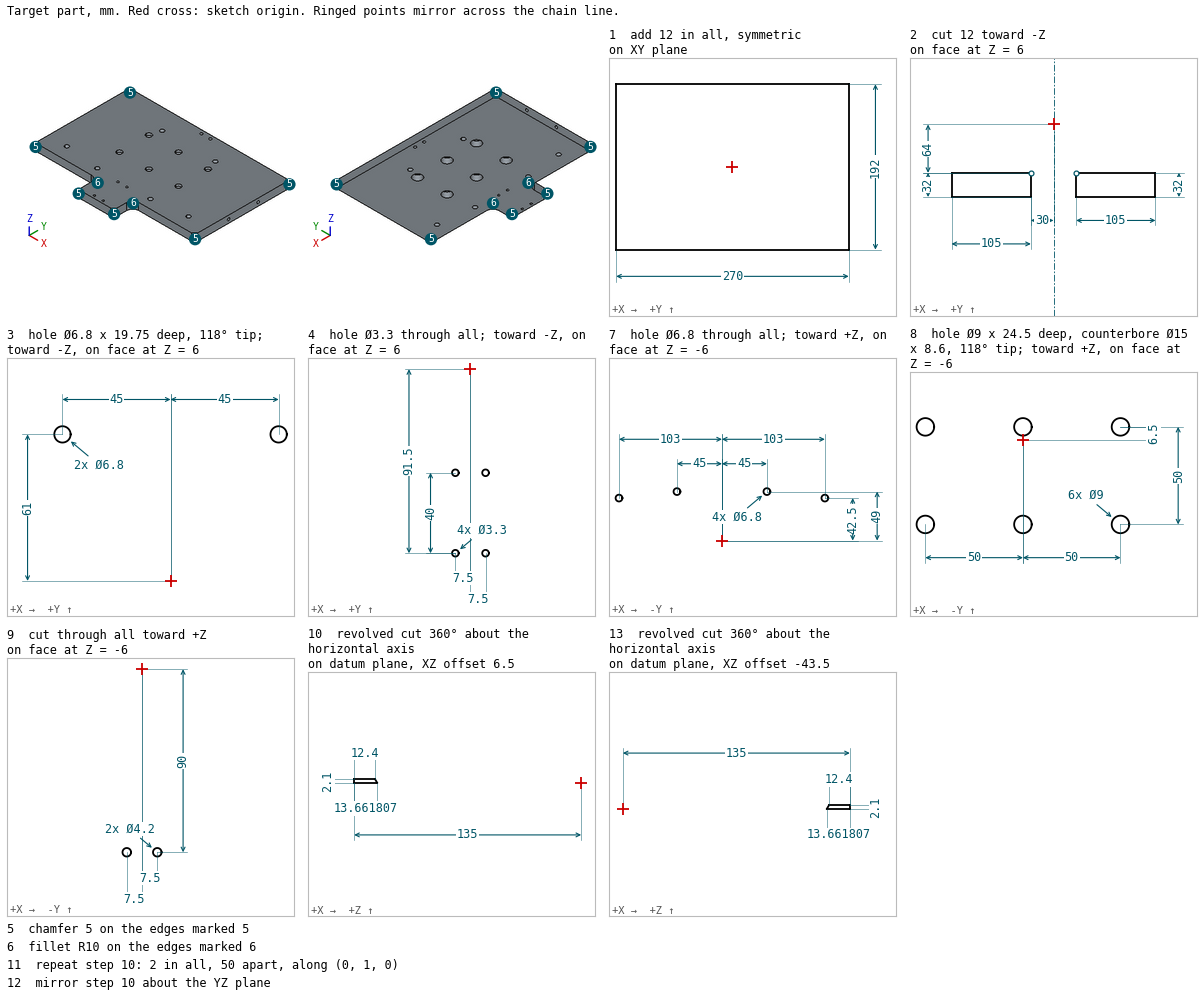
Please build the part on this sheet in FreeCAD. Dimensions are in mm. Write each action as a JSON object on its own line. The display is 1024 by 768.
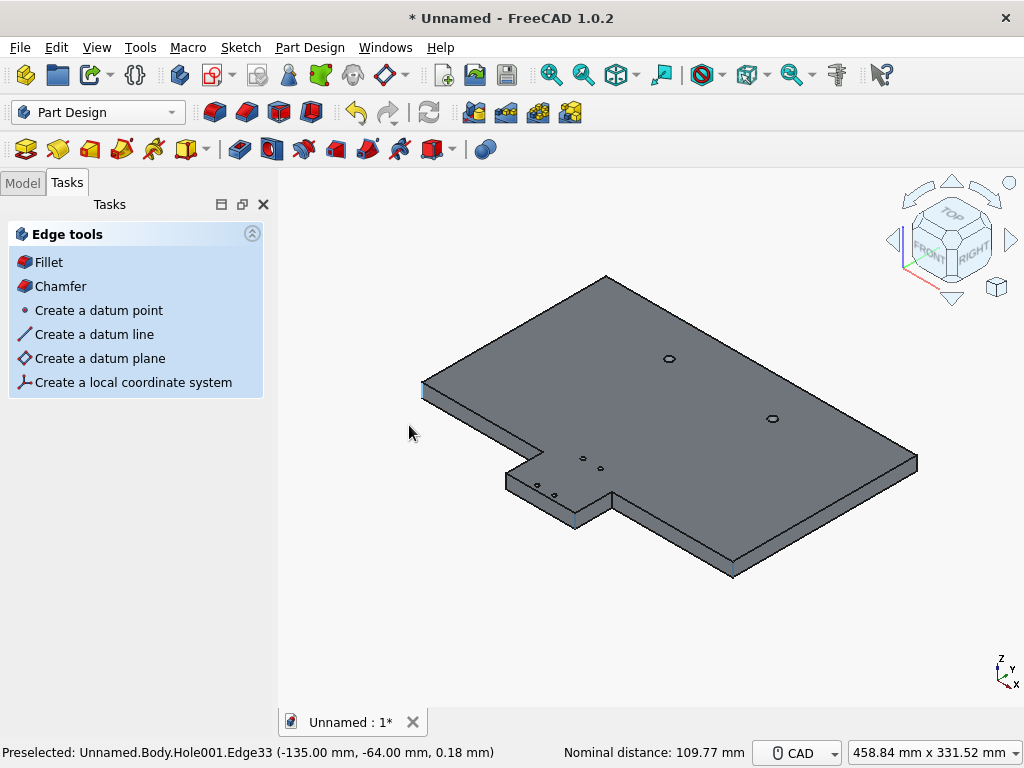
{"action": "scroll", "coordinate": [422, 389], "scroll_direction": "up", "scroll_amount": 4}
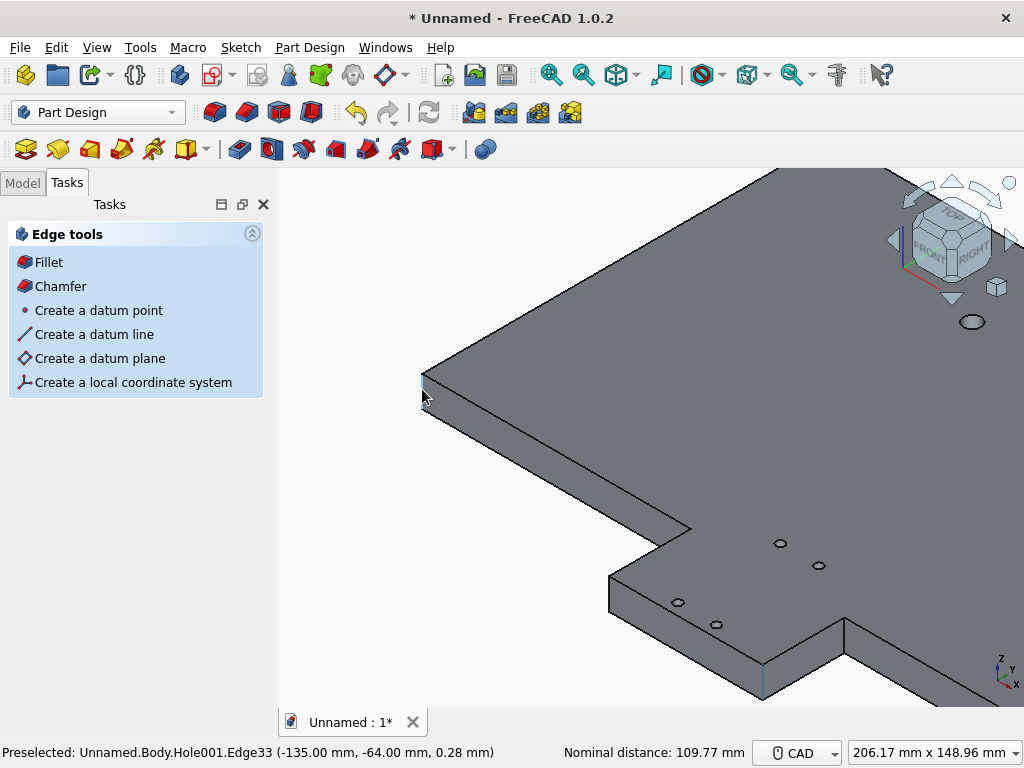
{"action": "key", "text": "v f"}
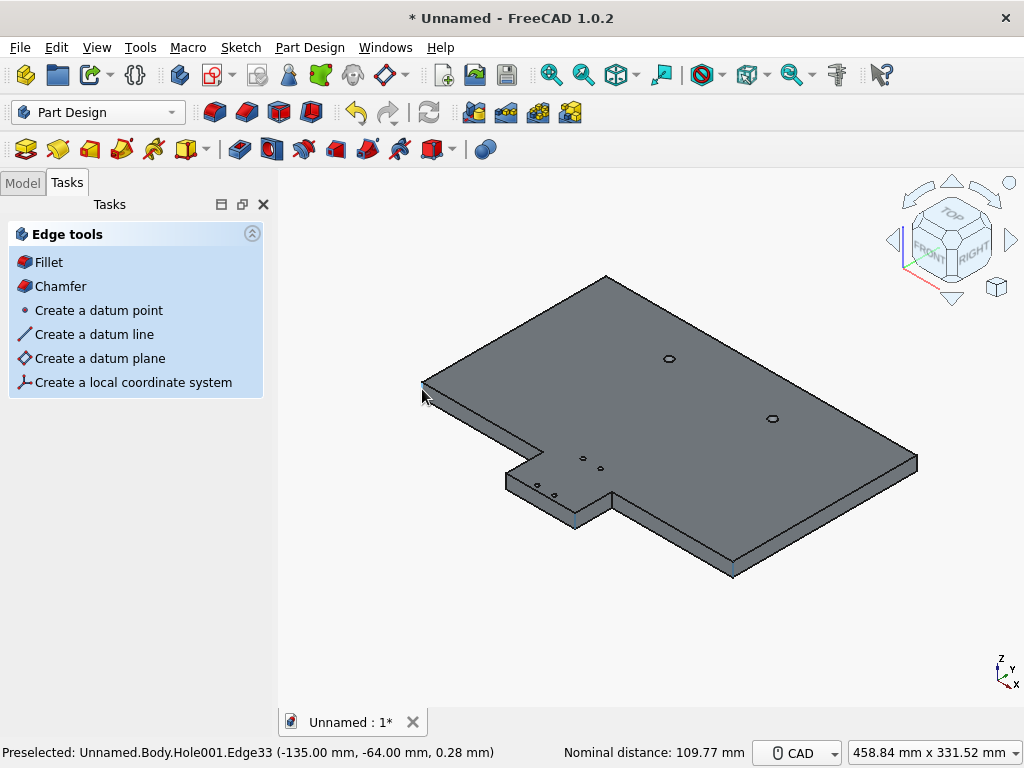
{"action": "key", "text": "2"}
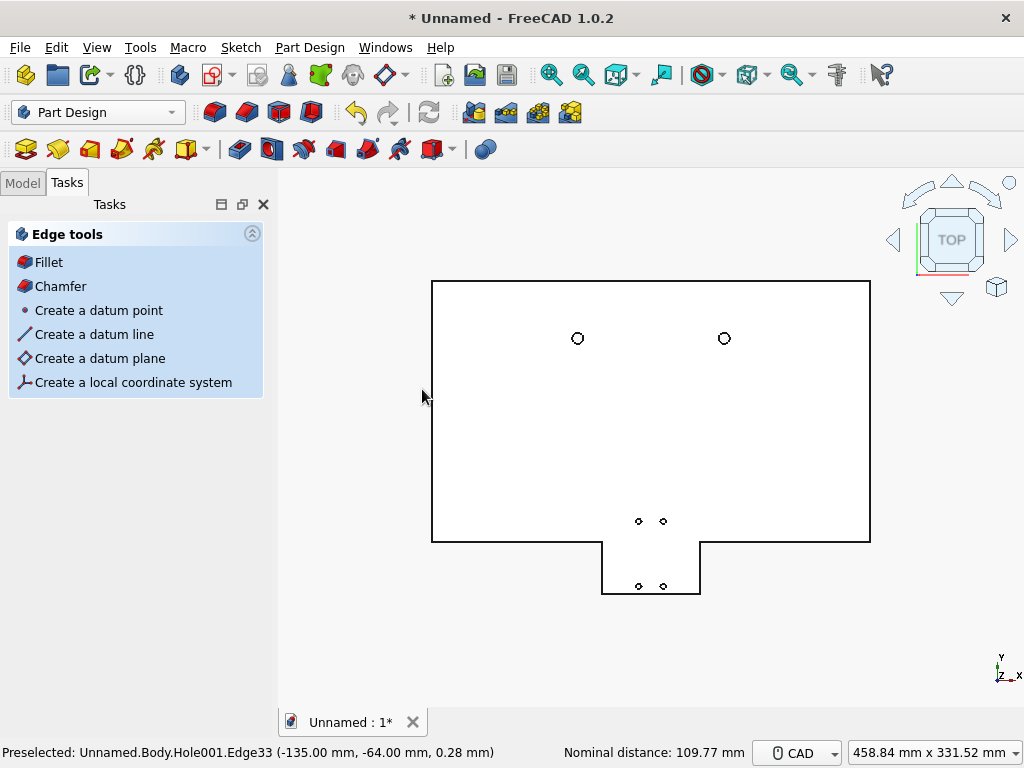
{"action": "scroll", "coordinate": [432, 541], "scroll_direction": "up", "scroll_amount": 4}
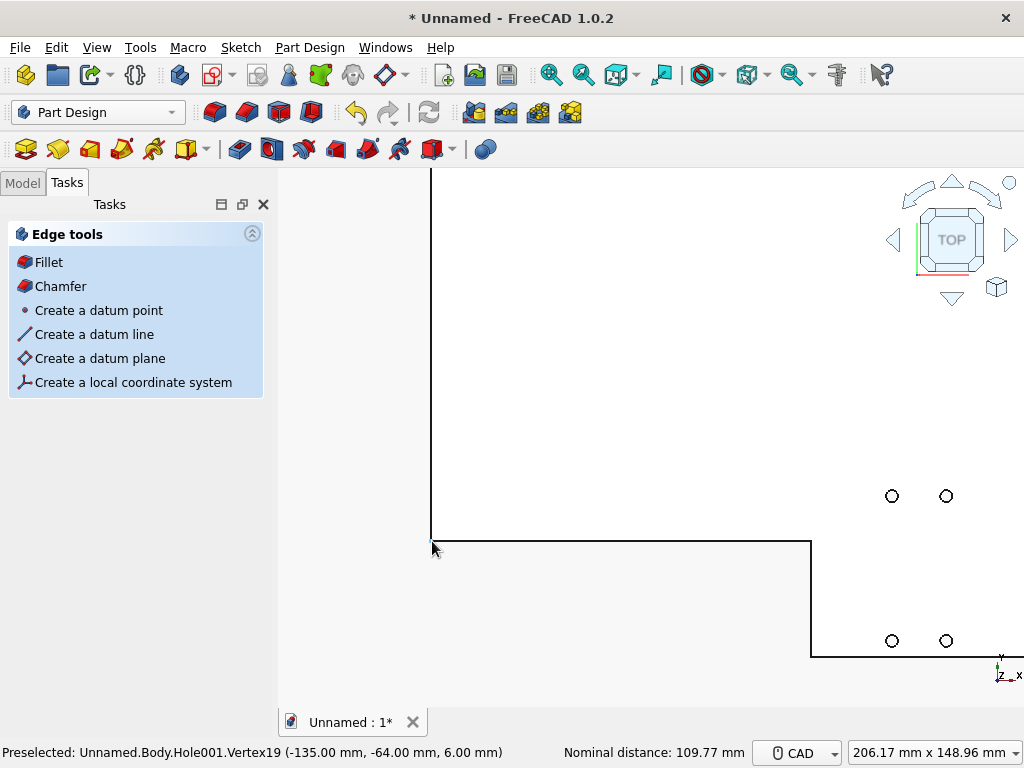
{"action": "key", "text": "v f"}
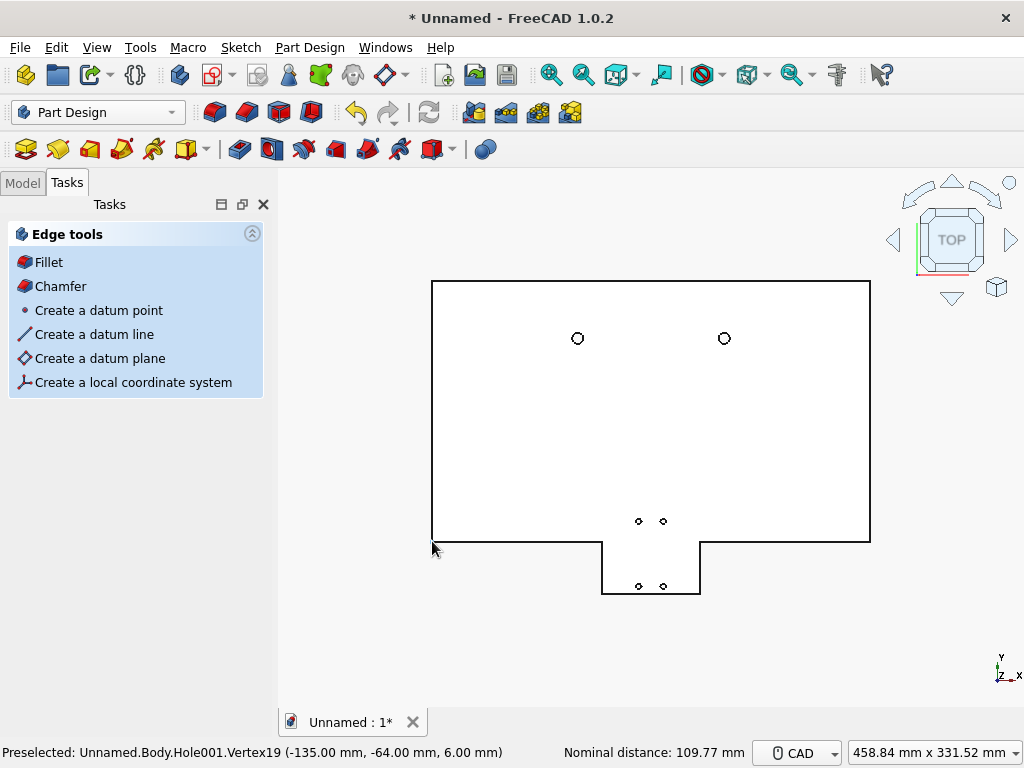
{"action": "key", "text": "1"}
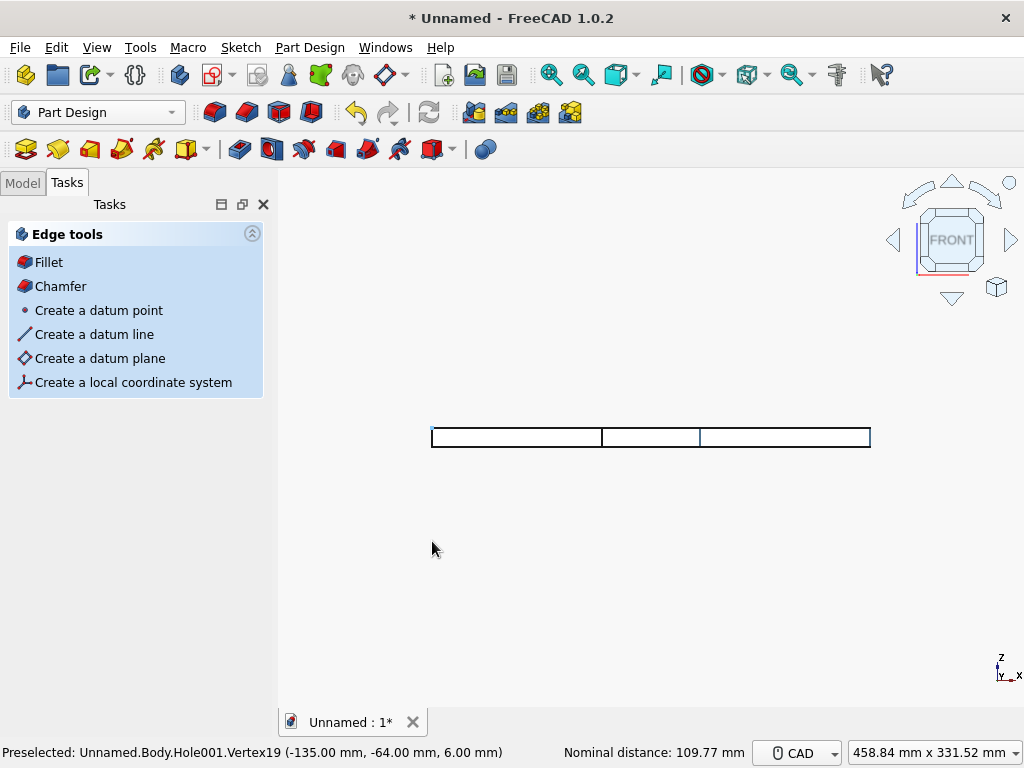
{"action": "left_click", "coordinate": [432, 436], "text": "ctrl"}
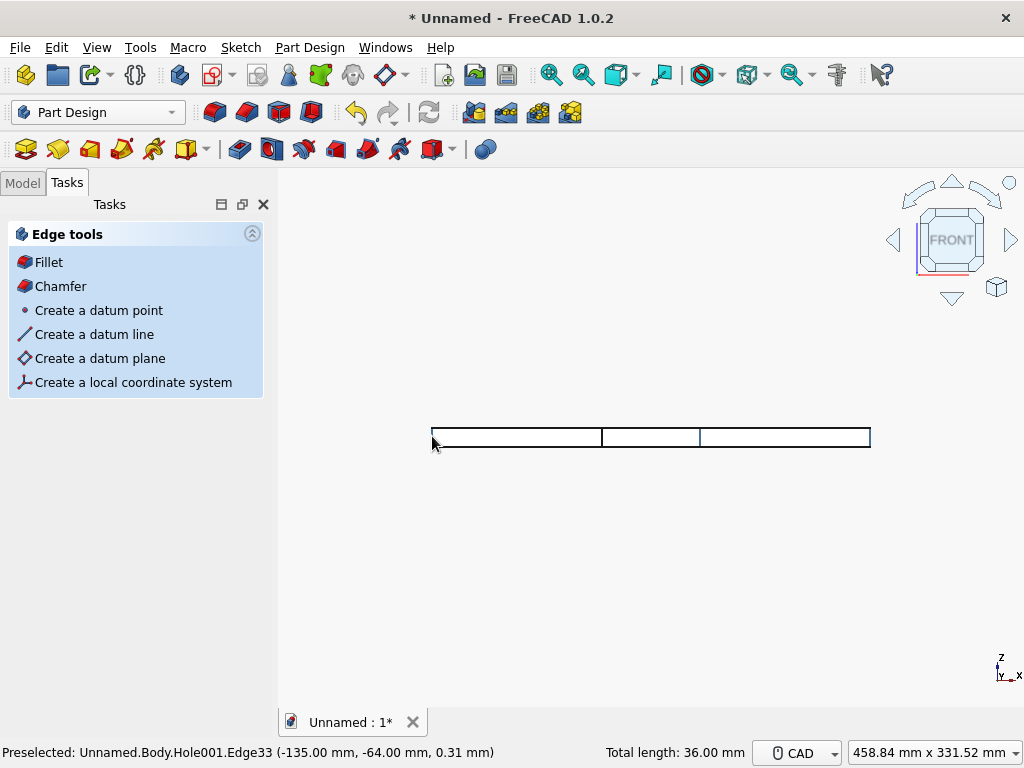
{"action": "left_click", "coordinate": [602, 436], "text": "ctrl"}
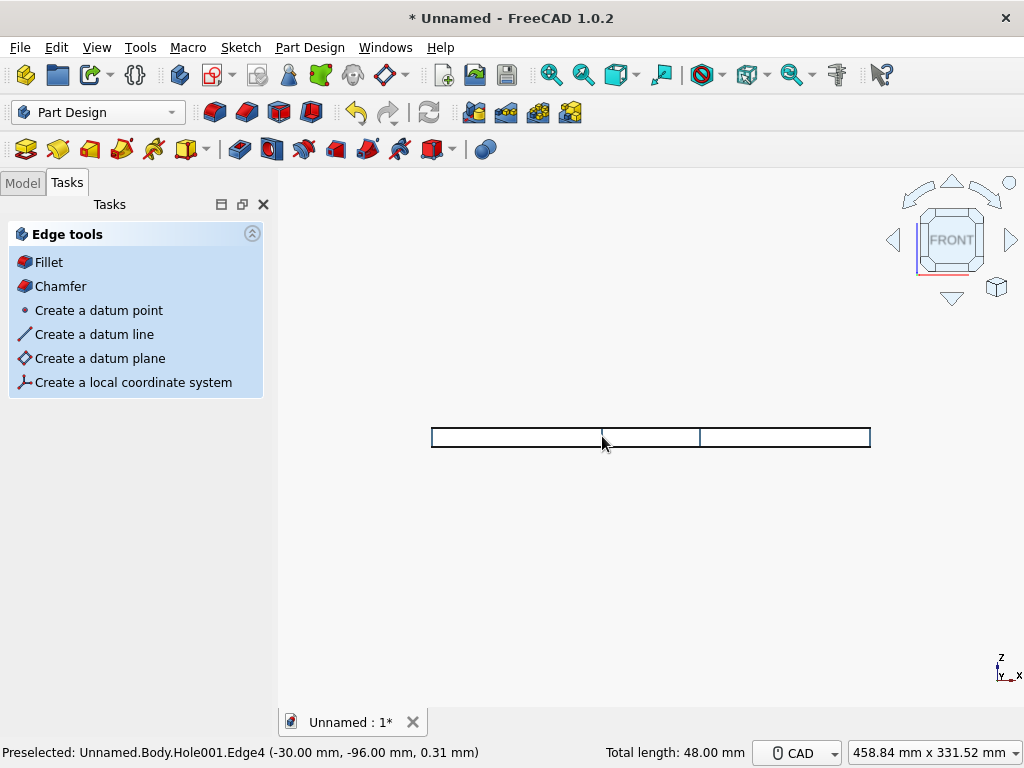
{"action": "scroll", "coordinate": [432, 436], "scroll_direction": "up", "scroll_amount": 4}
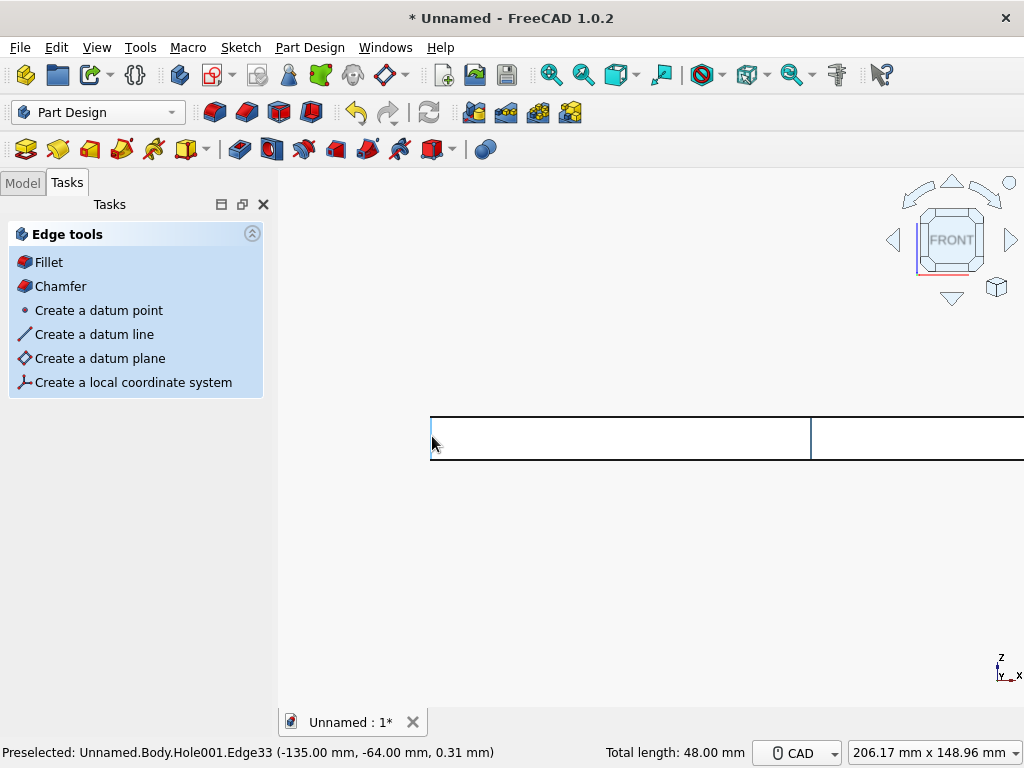
{"action": "left_click", "coordinate": [552, 76]}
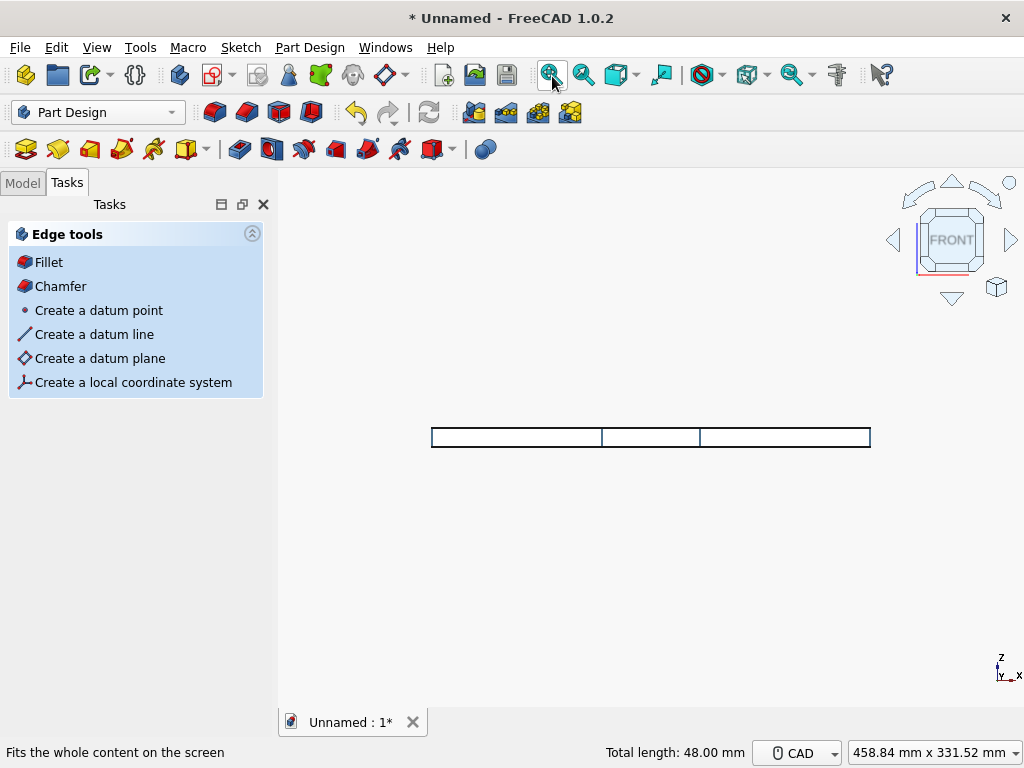
{"action": "key", "text": "3"}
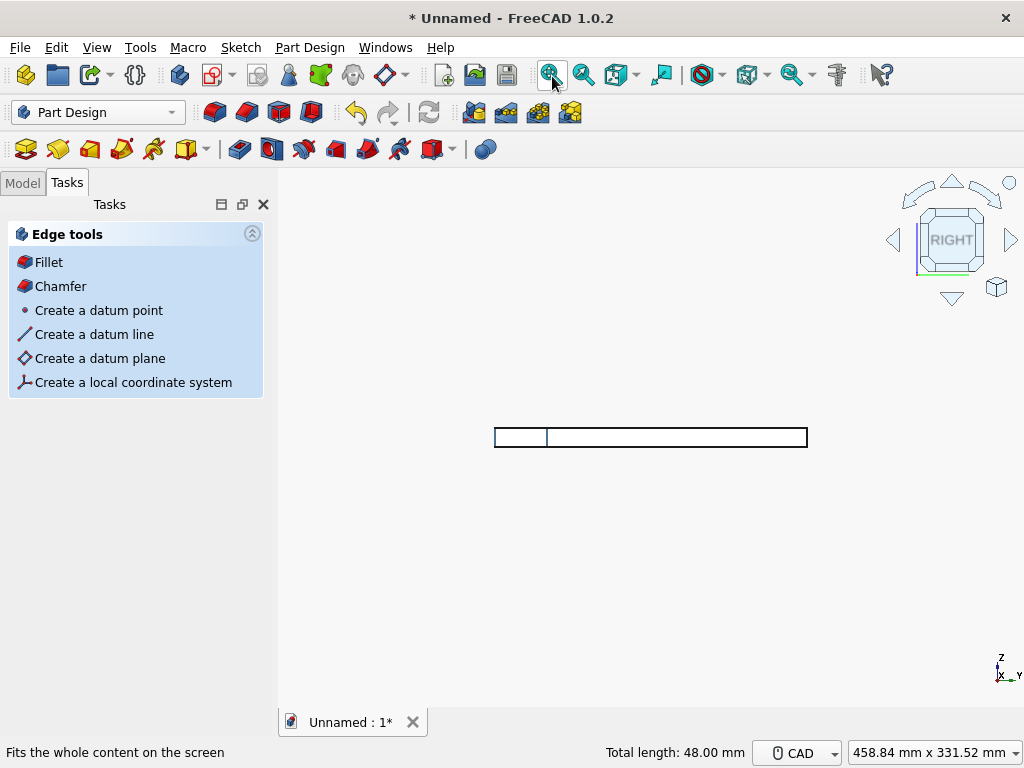
{"action": "left_click", "coordinate": [552, 76]}